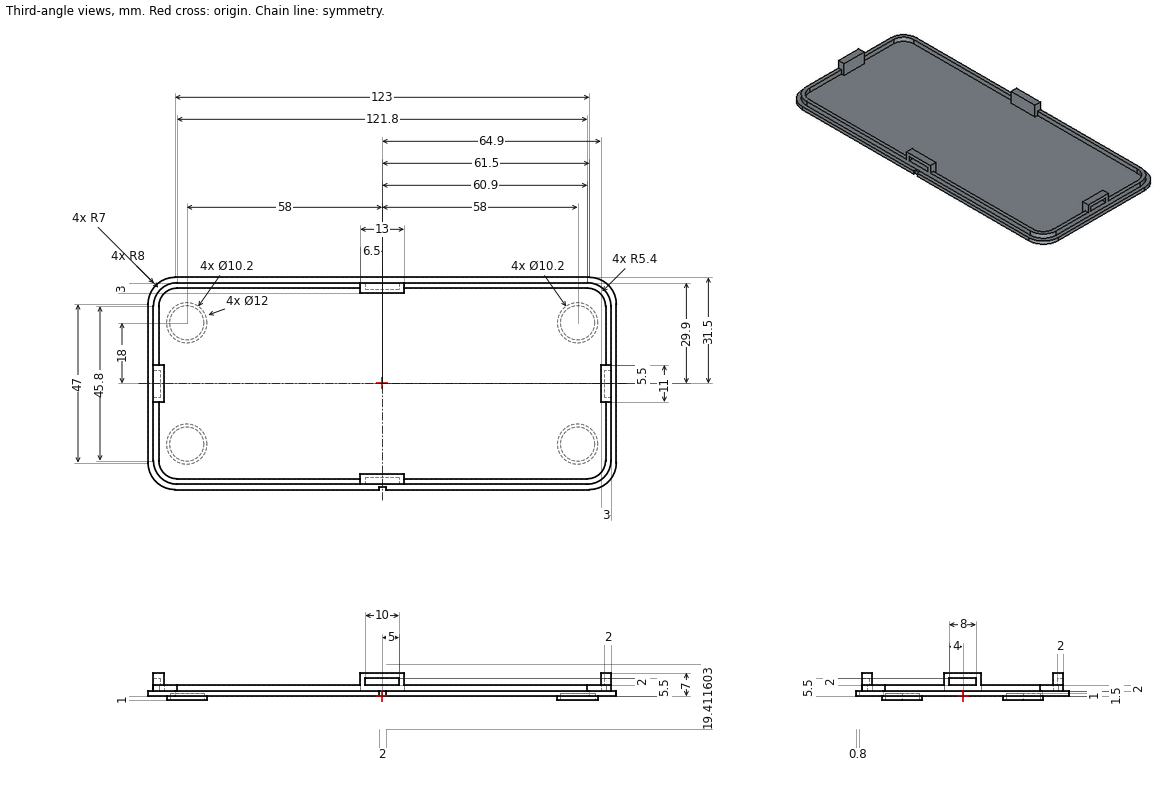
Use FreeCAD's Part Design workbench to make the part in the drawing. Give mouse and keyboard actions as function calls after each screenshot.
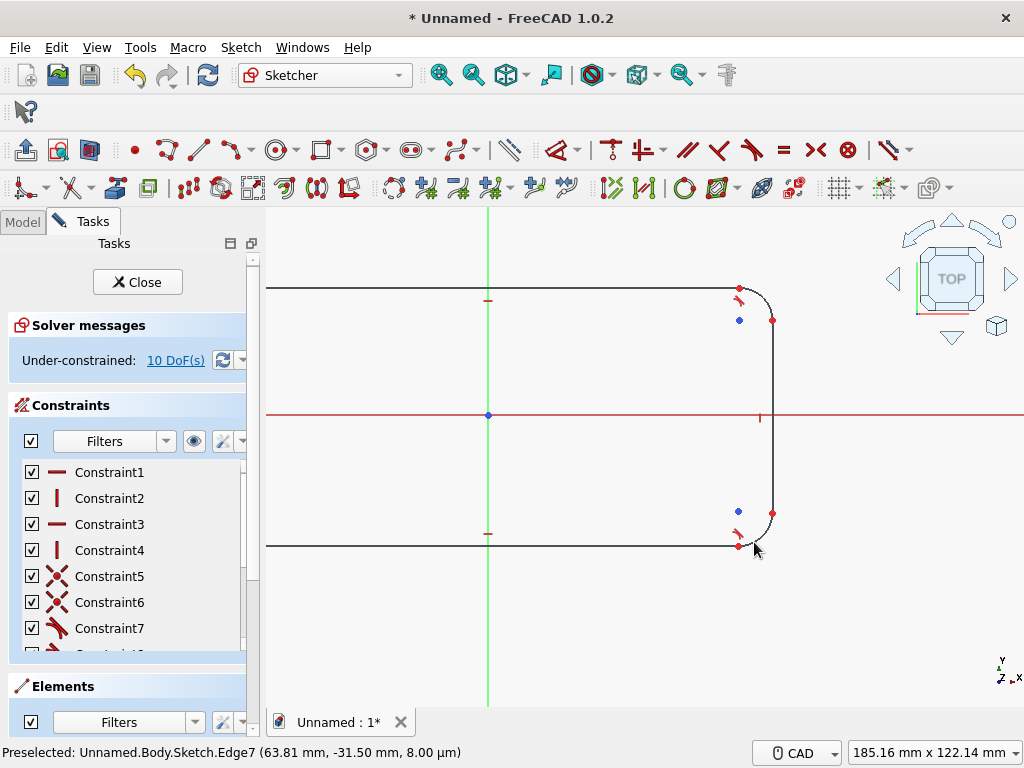
click(773, 456)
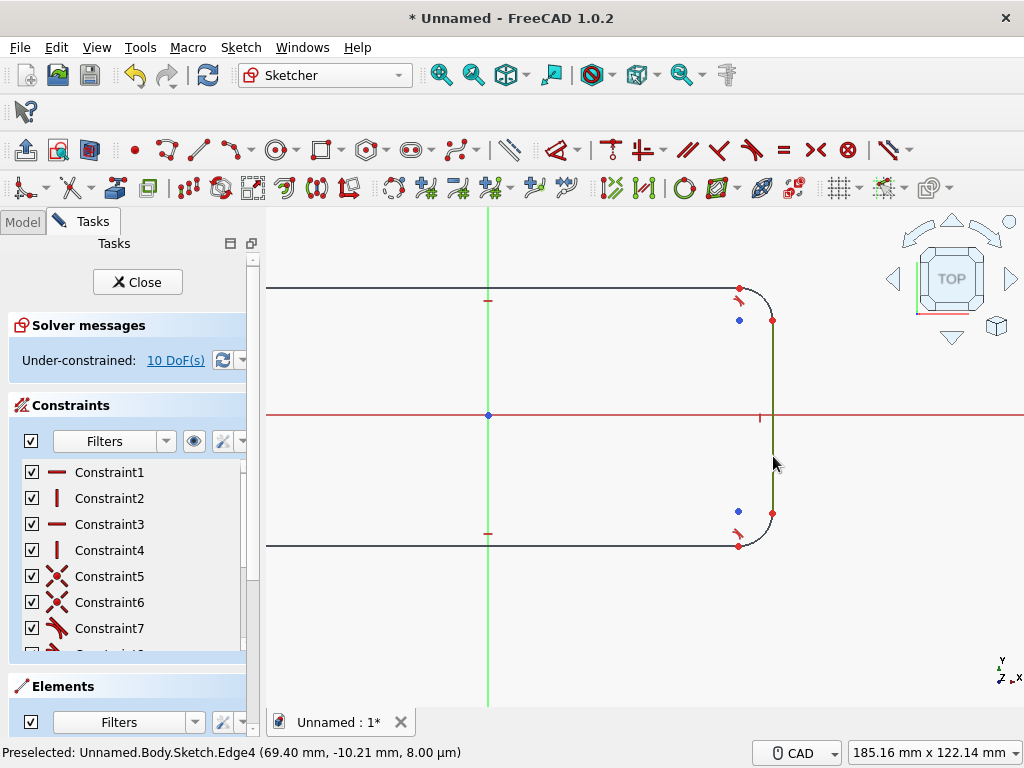
click(753, 543)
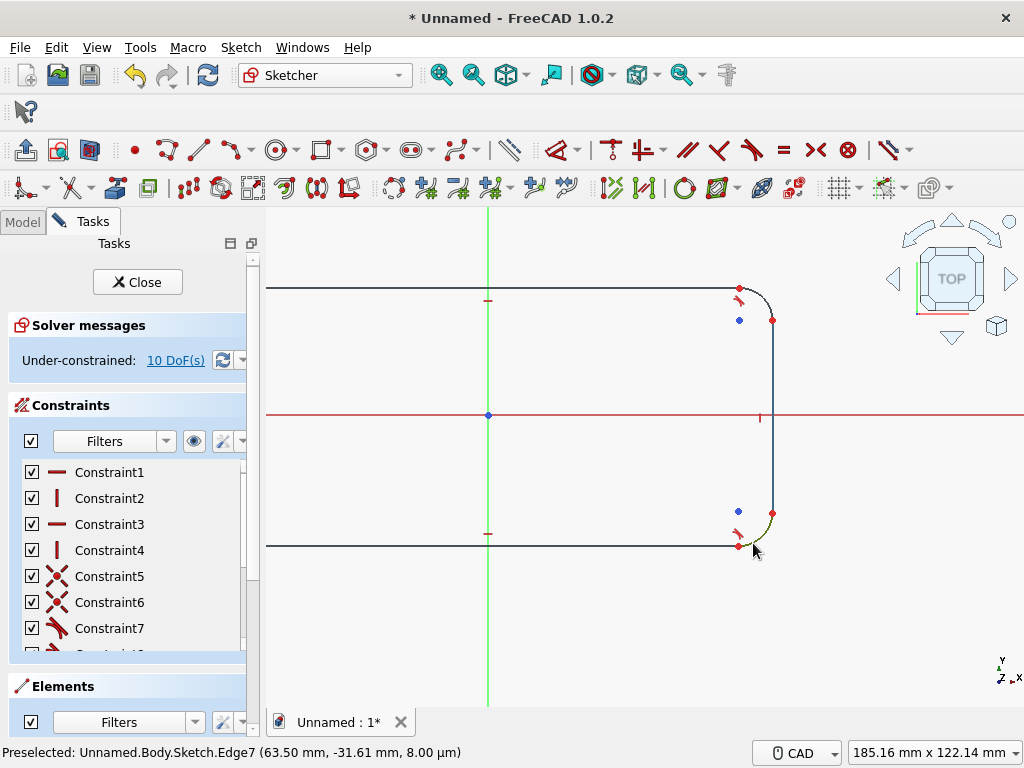
key(t)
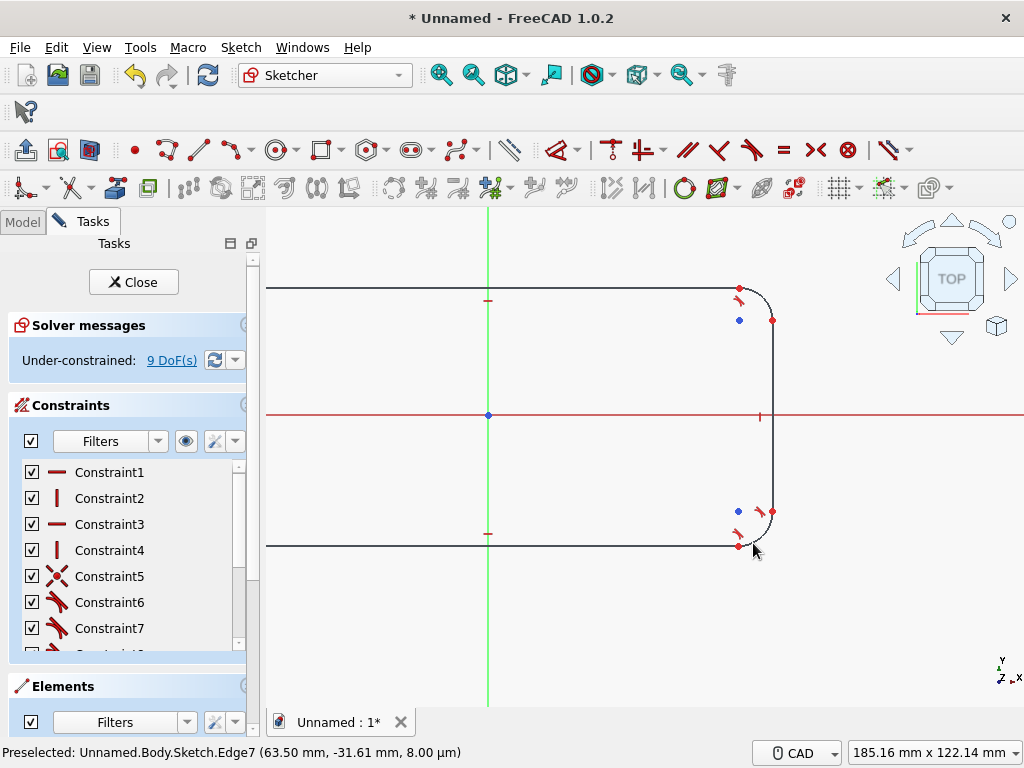
click(773, 454)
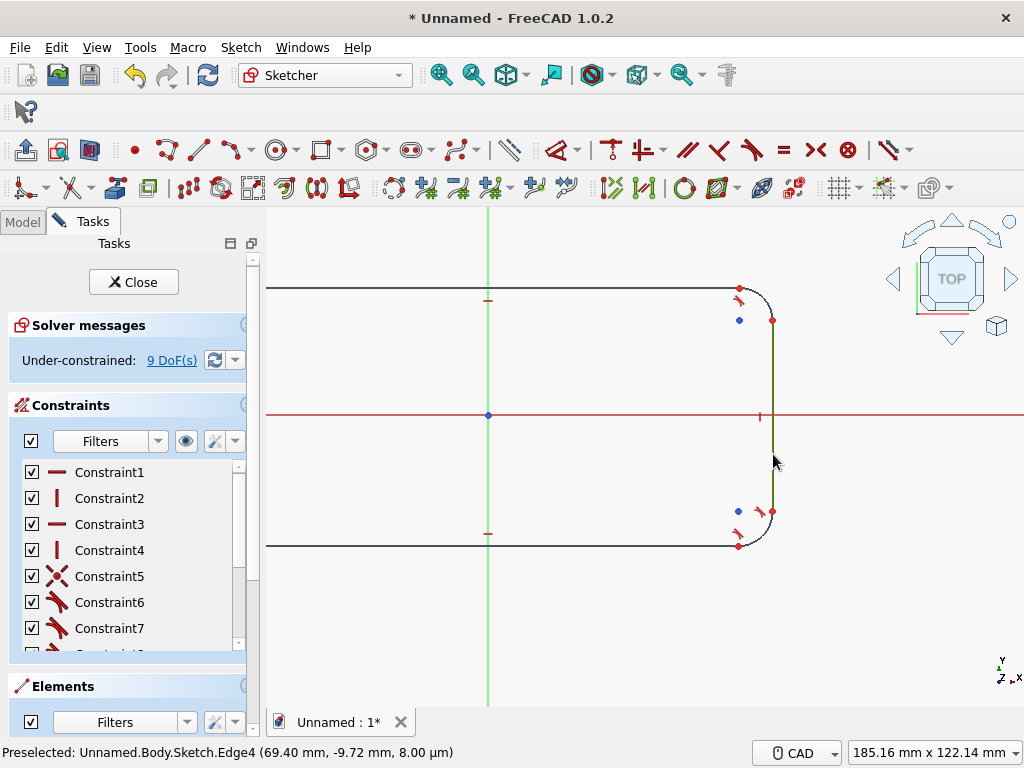
click(769, 306)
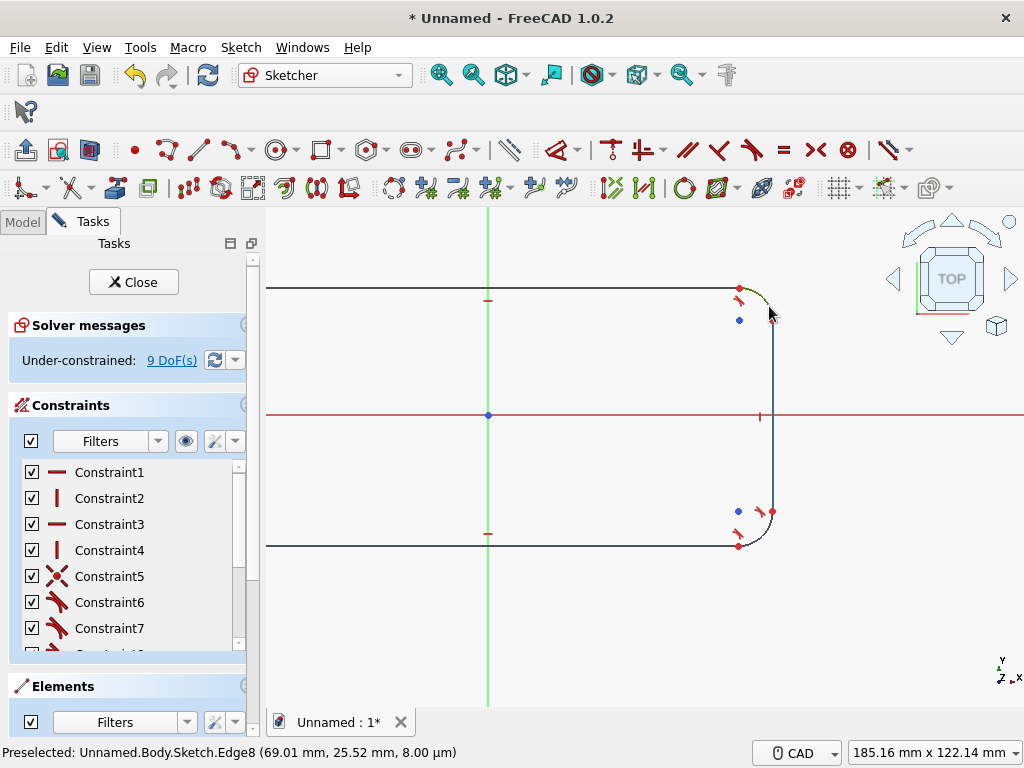
click(752, 150)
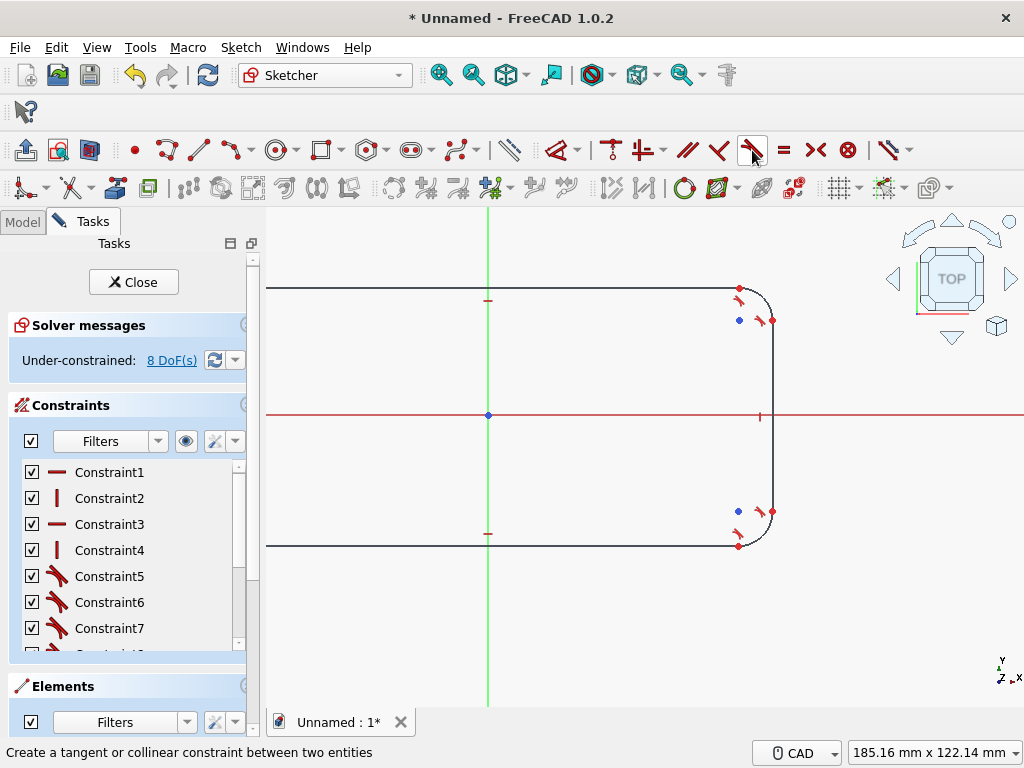
scroll(756, 542, down, 2)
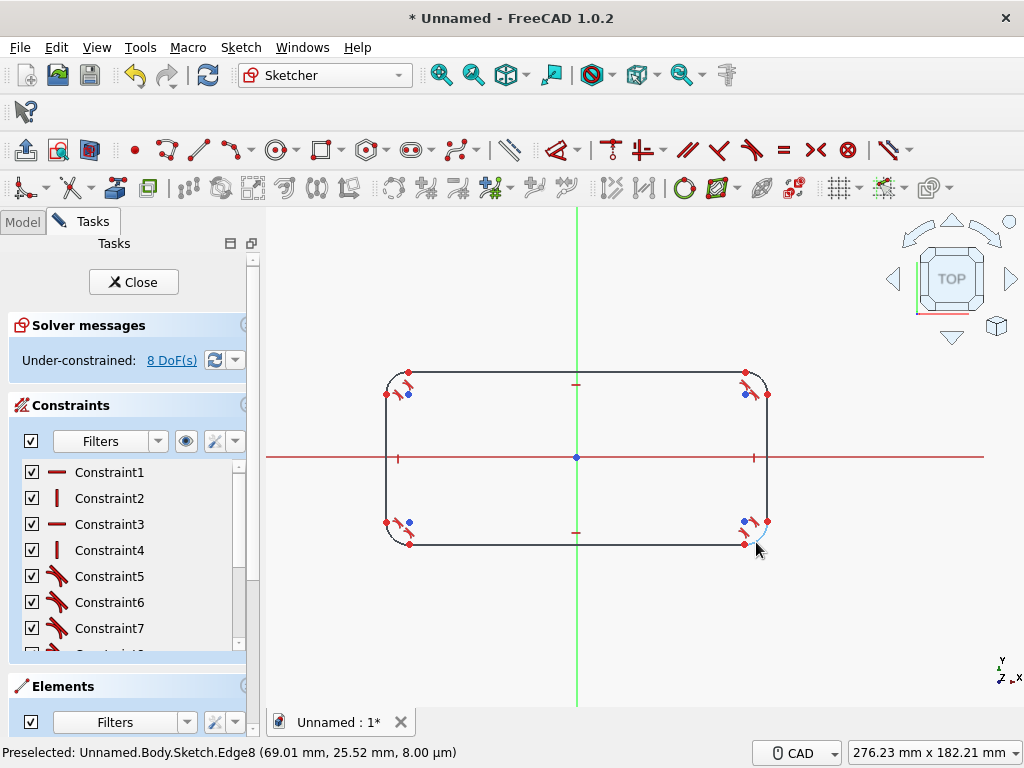
scroll(398, 374, up, 2)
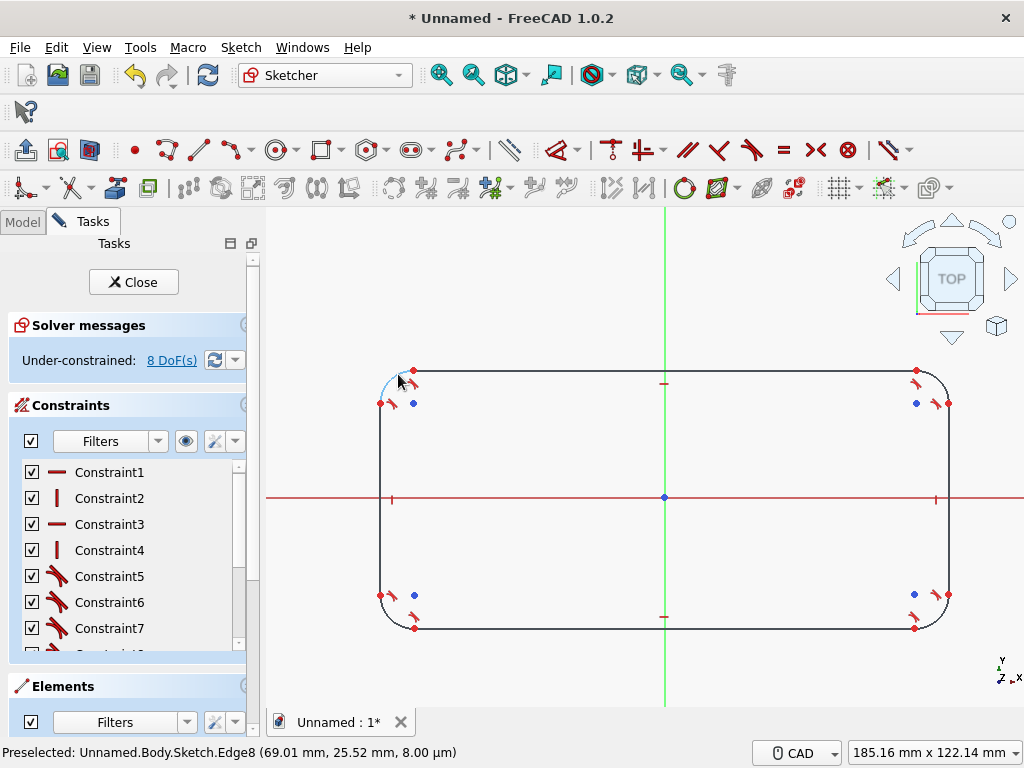
click(398, 374)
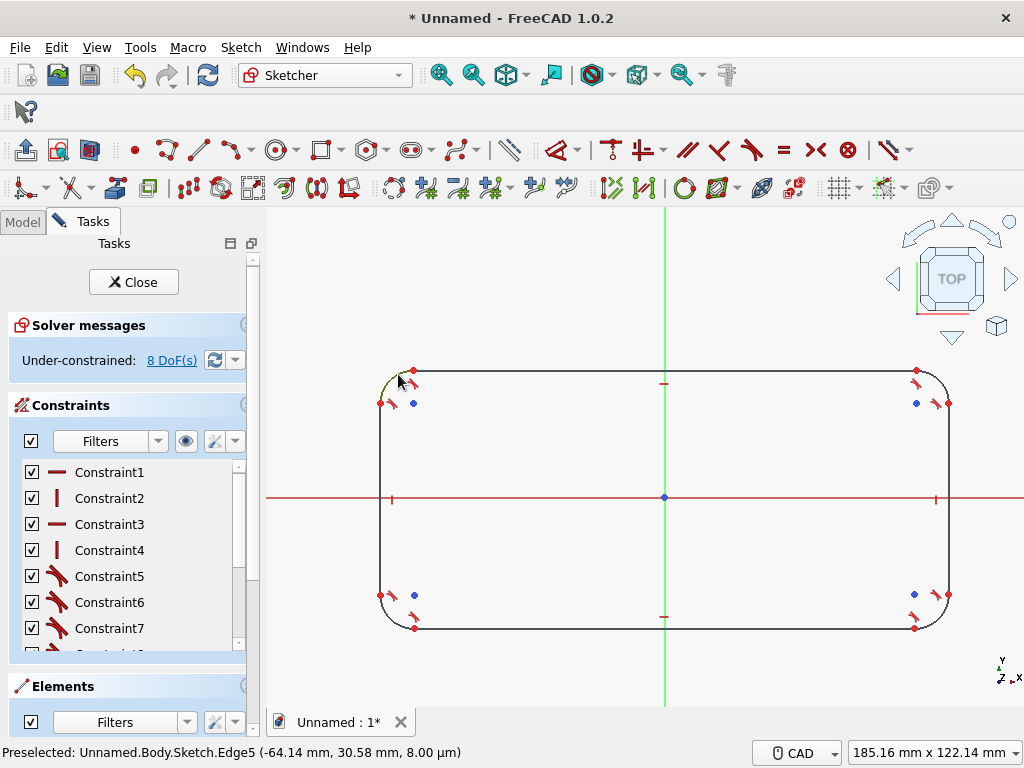
click(384, 610)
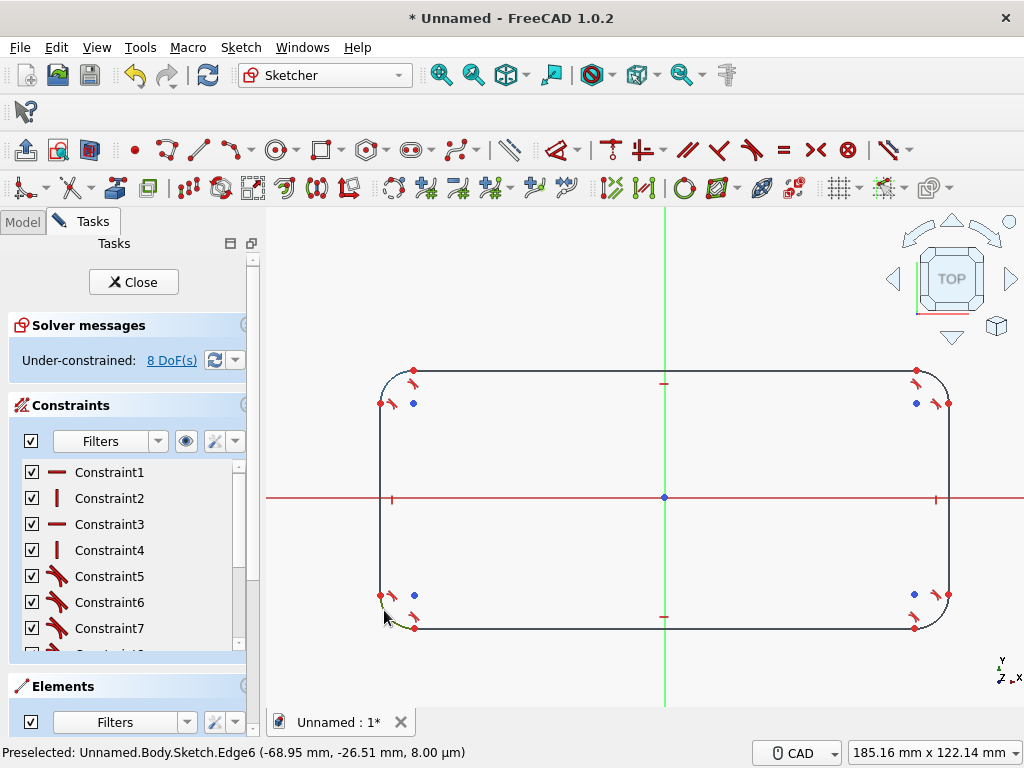
scroll(397, 374, down, 2)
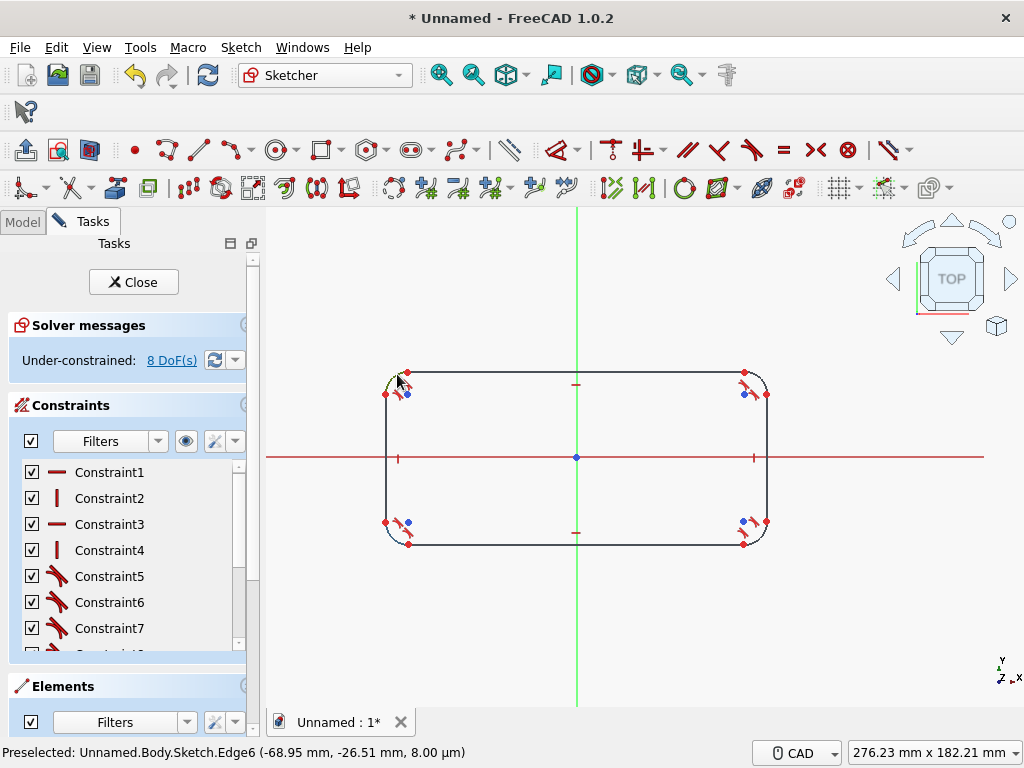
scroll(754, 542, up, 2)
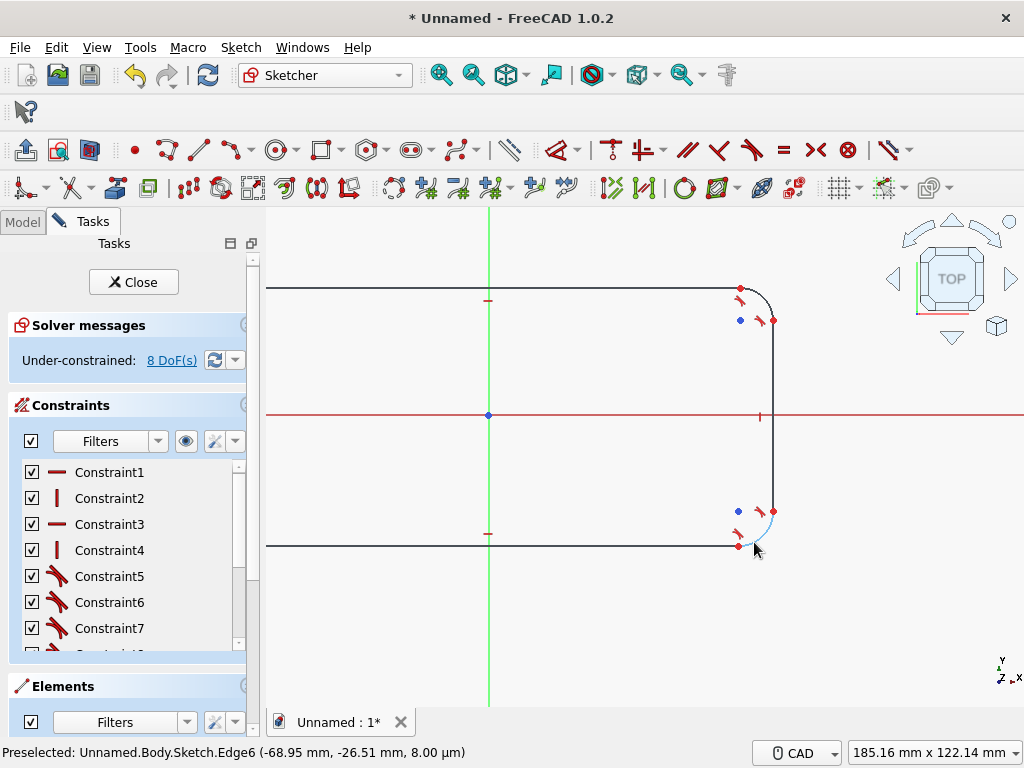
click(754, 542)